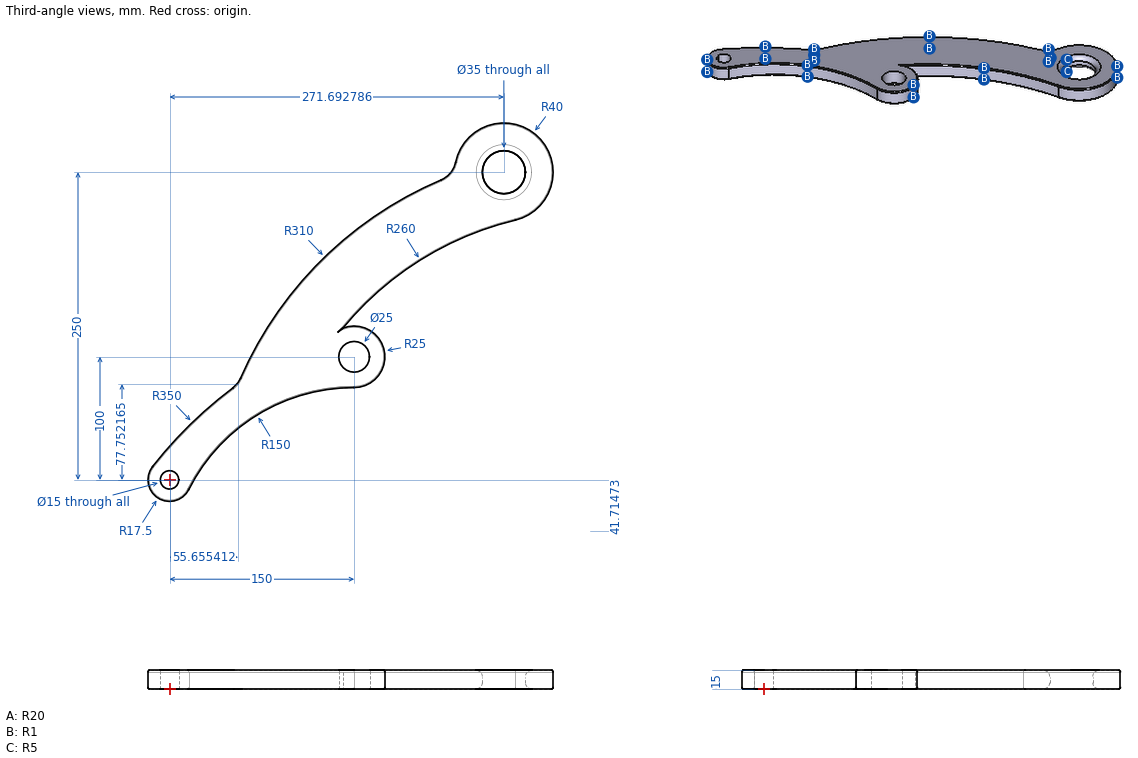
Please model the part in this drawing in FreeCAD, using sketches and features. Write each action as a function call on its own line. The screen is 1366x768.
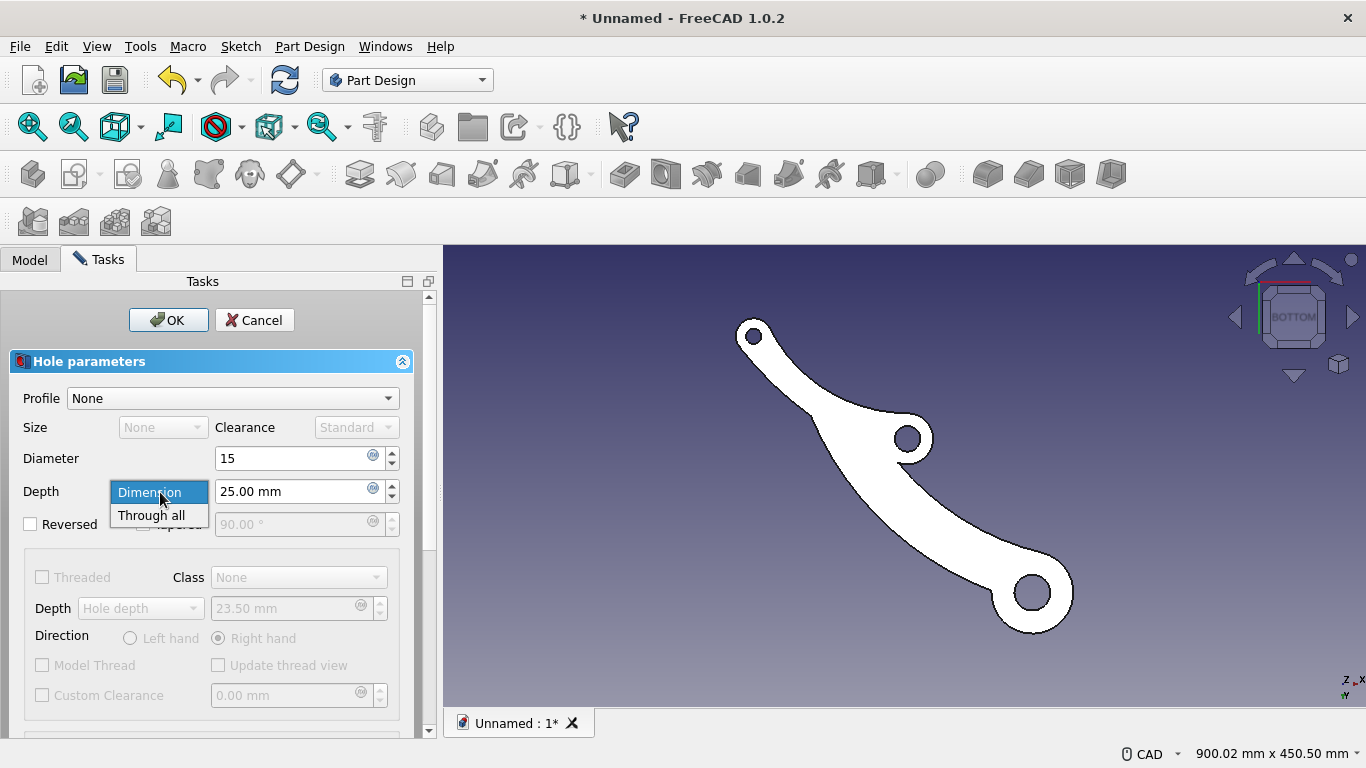
click(158, 516)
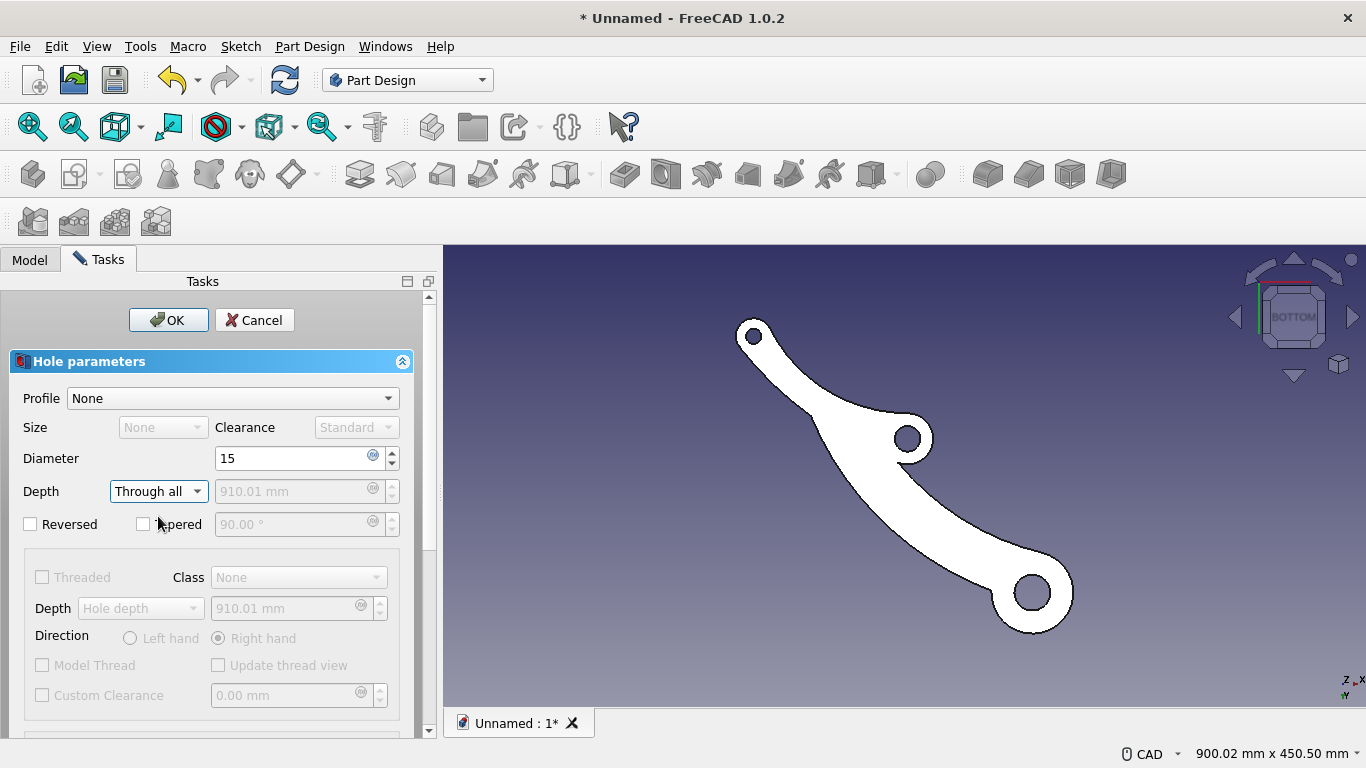
click(169, 320)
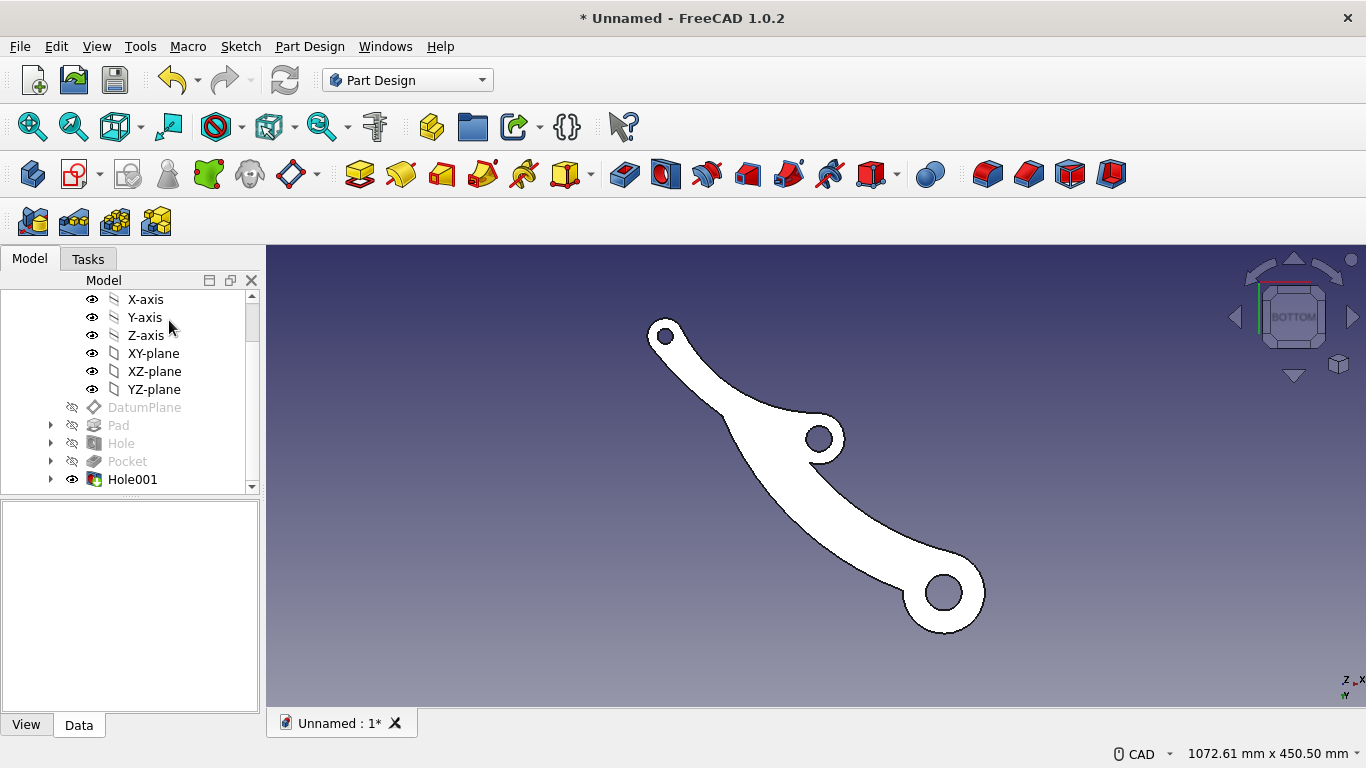
scroll(722, 415, up, 5)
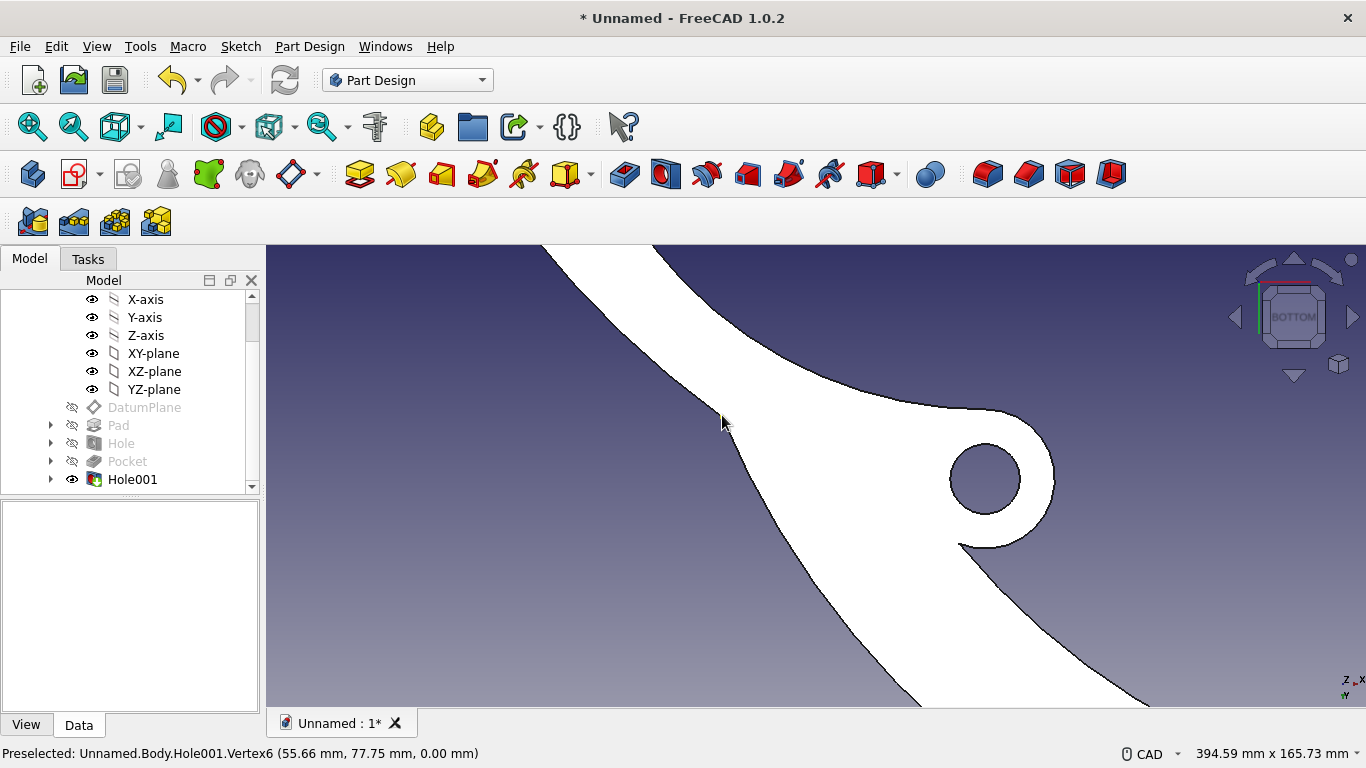
key(v)
key(f)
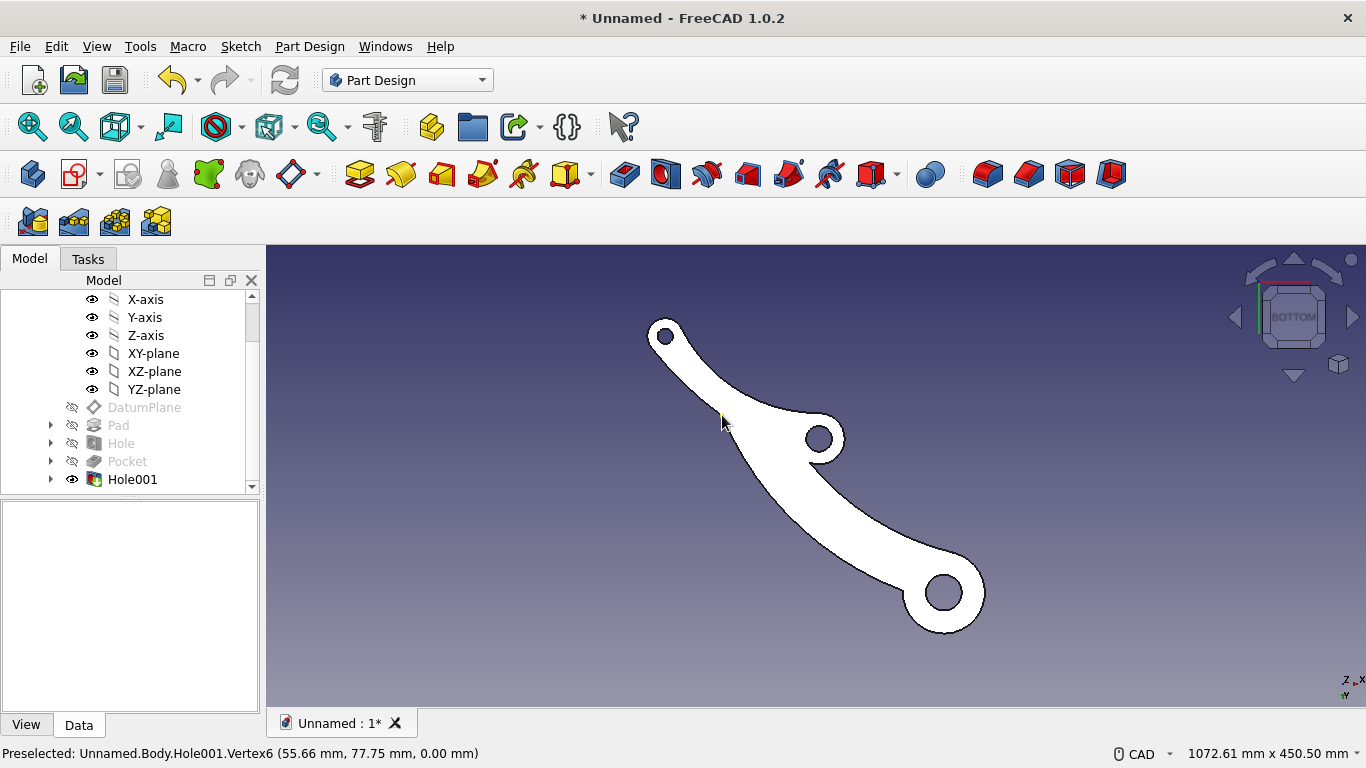
key(0)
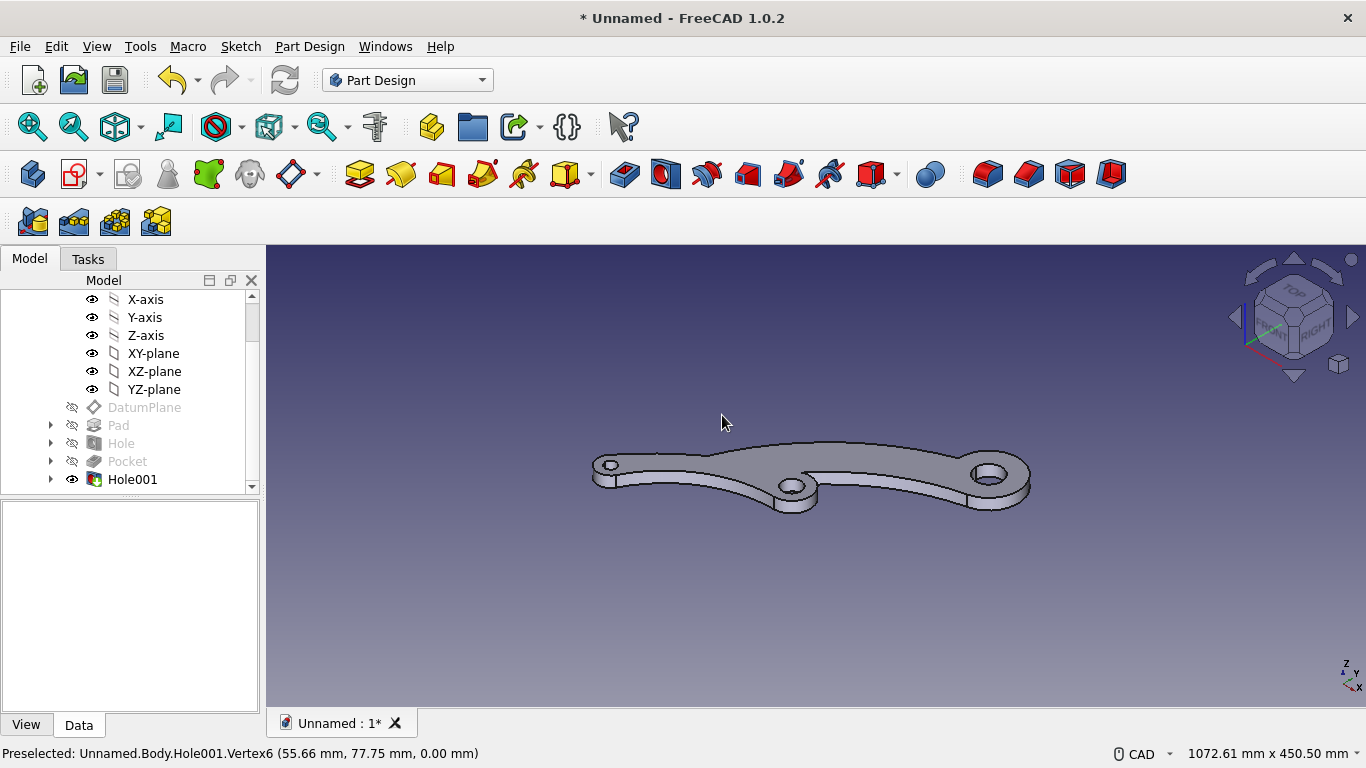
scroll(707, 461, up, 5)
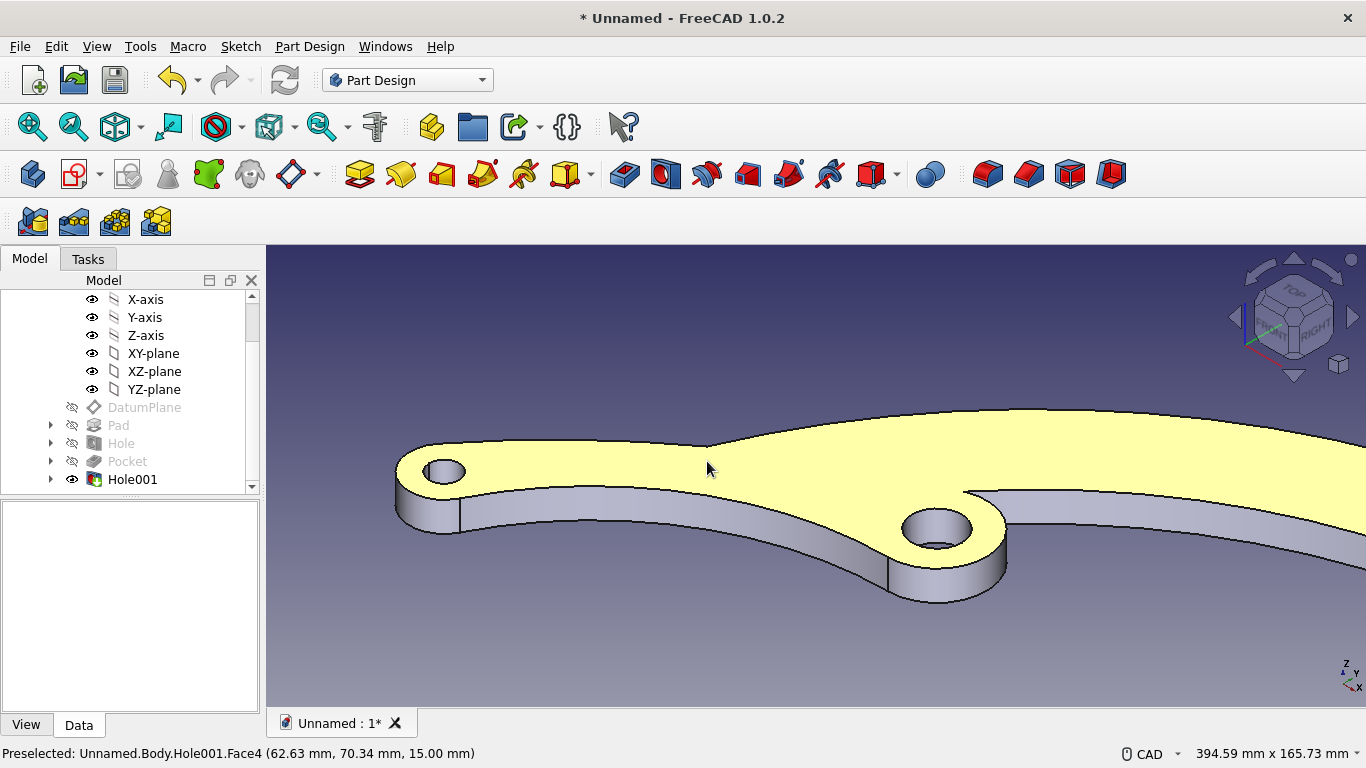
key(v)
key(f)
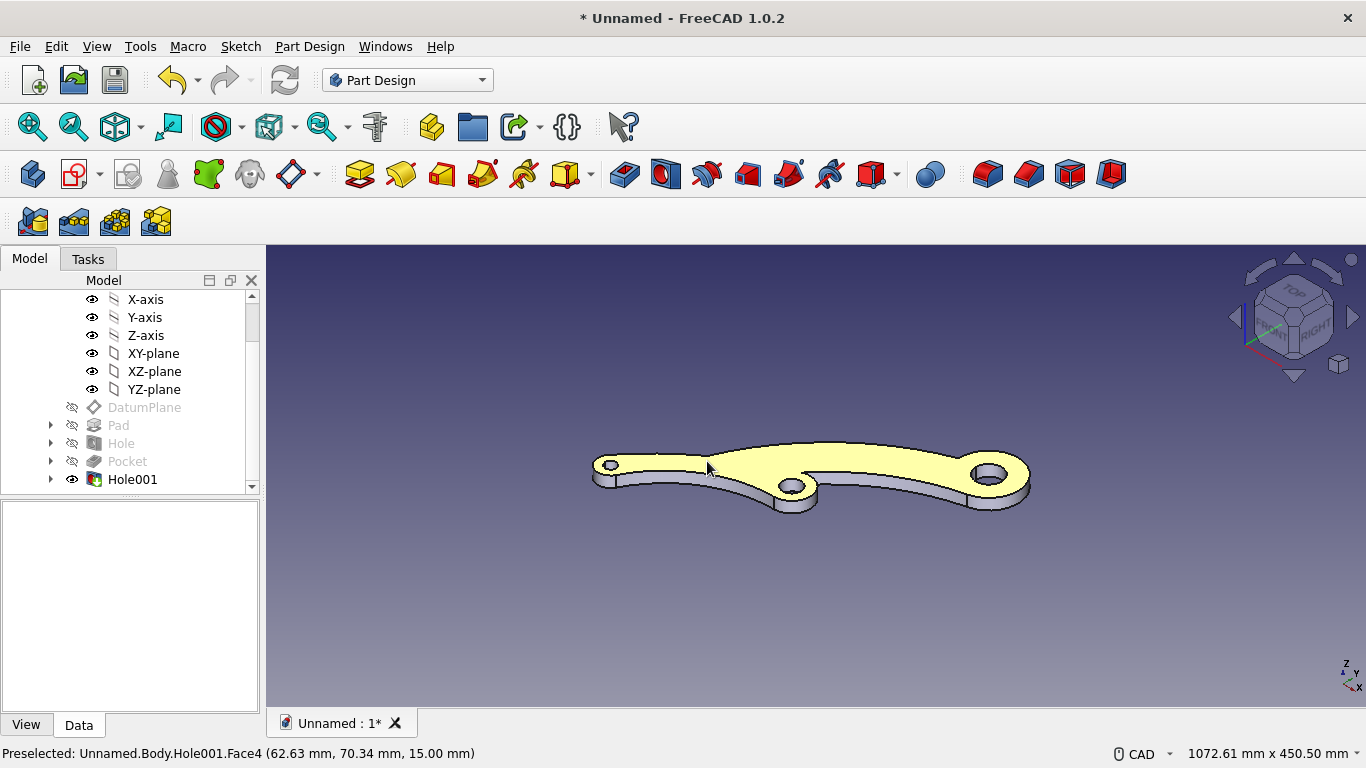
key(2)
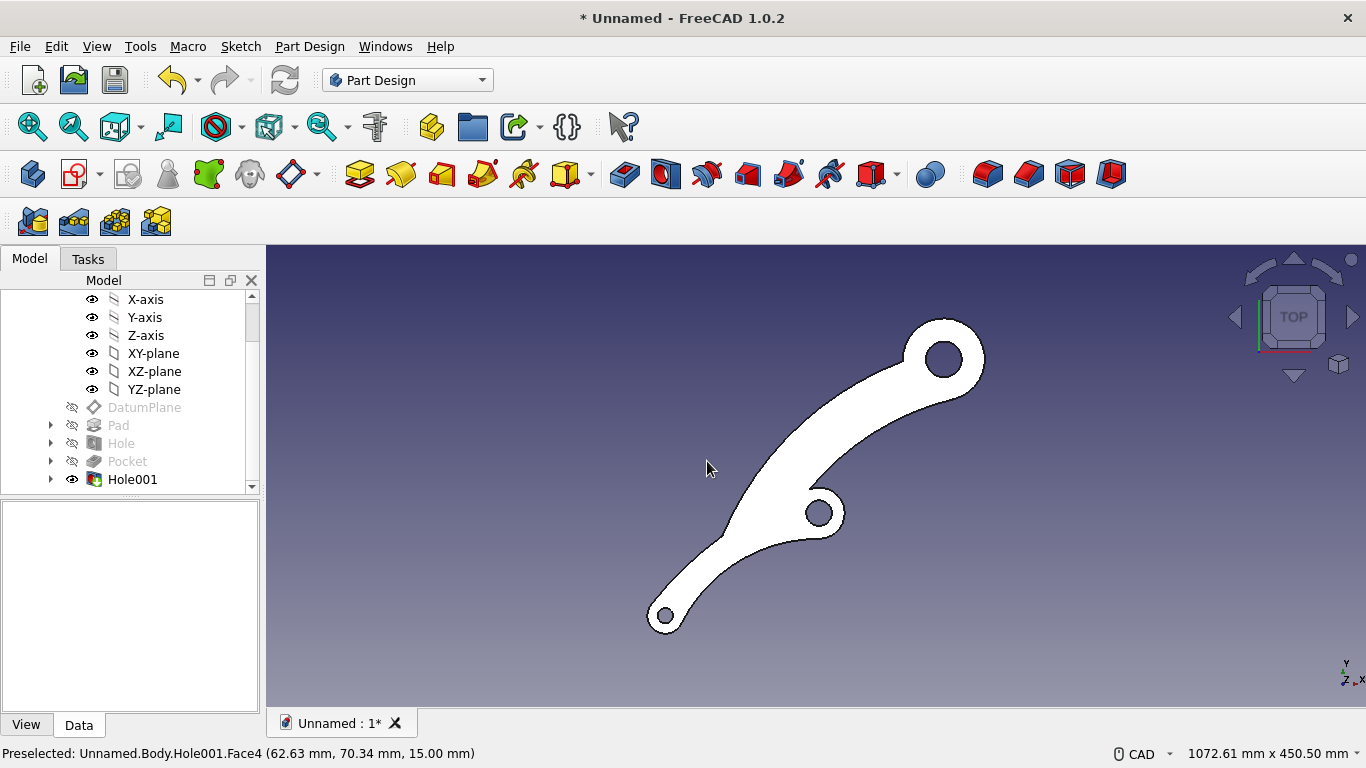
scroll(722, 535, up, 5)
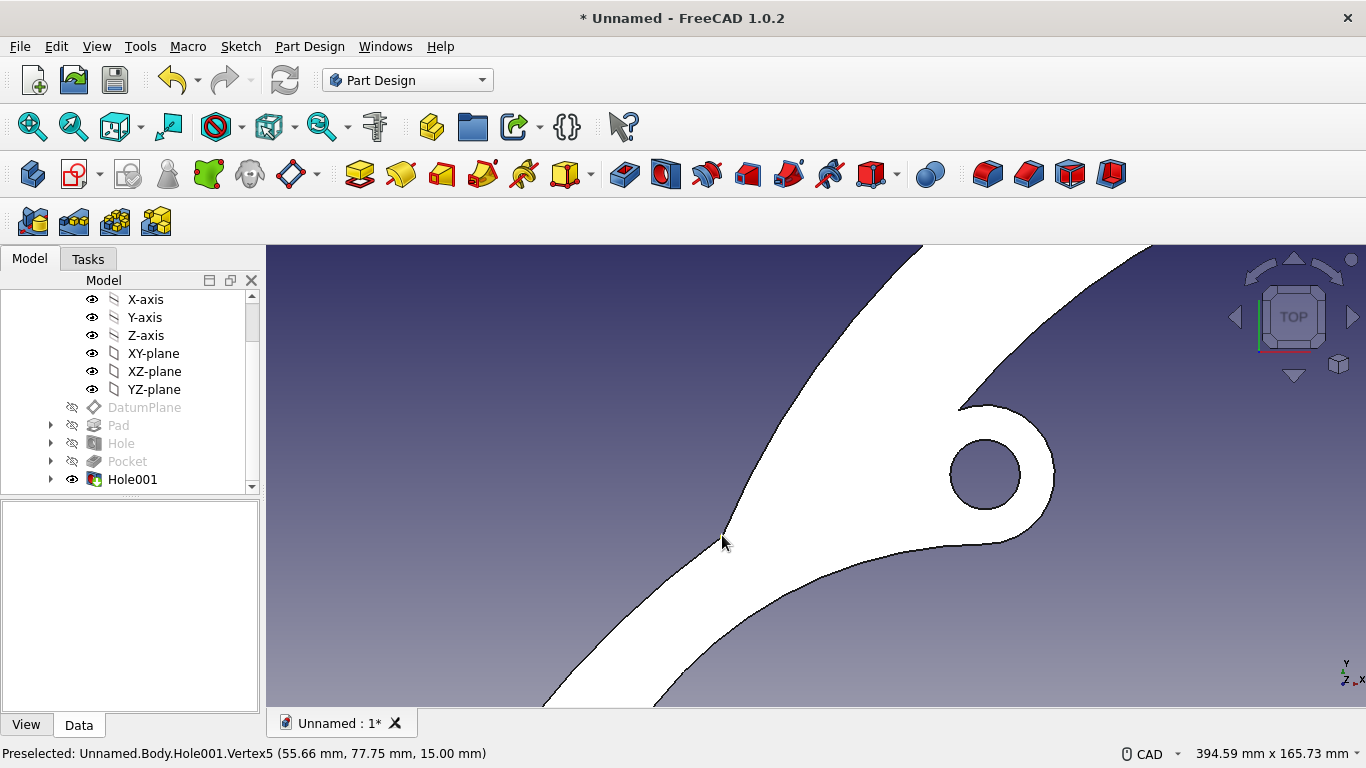
key(v)
key(f)